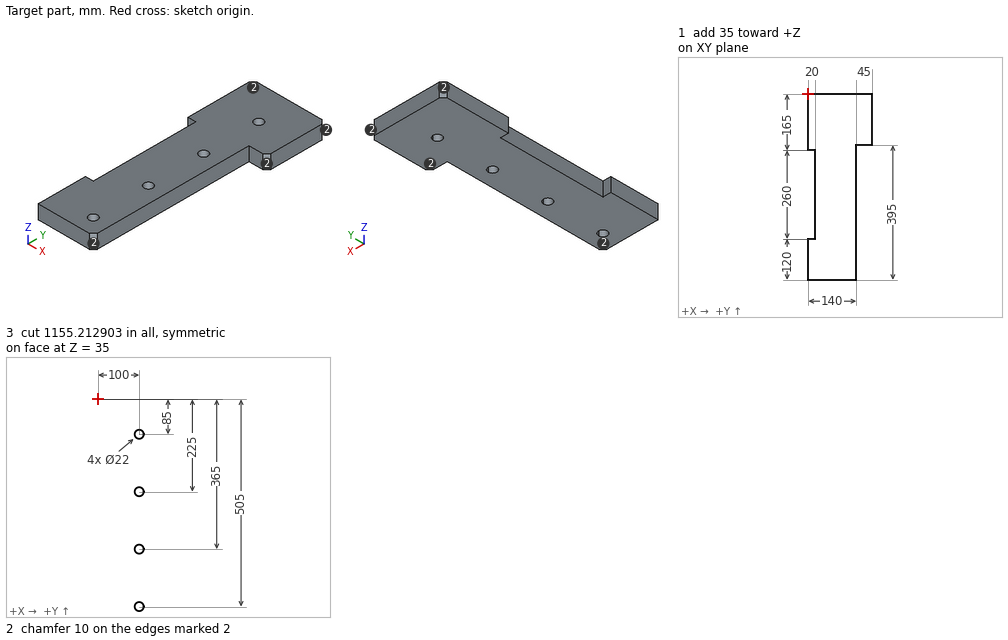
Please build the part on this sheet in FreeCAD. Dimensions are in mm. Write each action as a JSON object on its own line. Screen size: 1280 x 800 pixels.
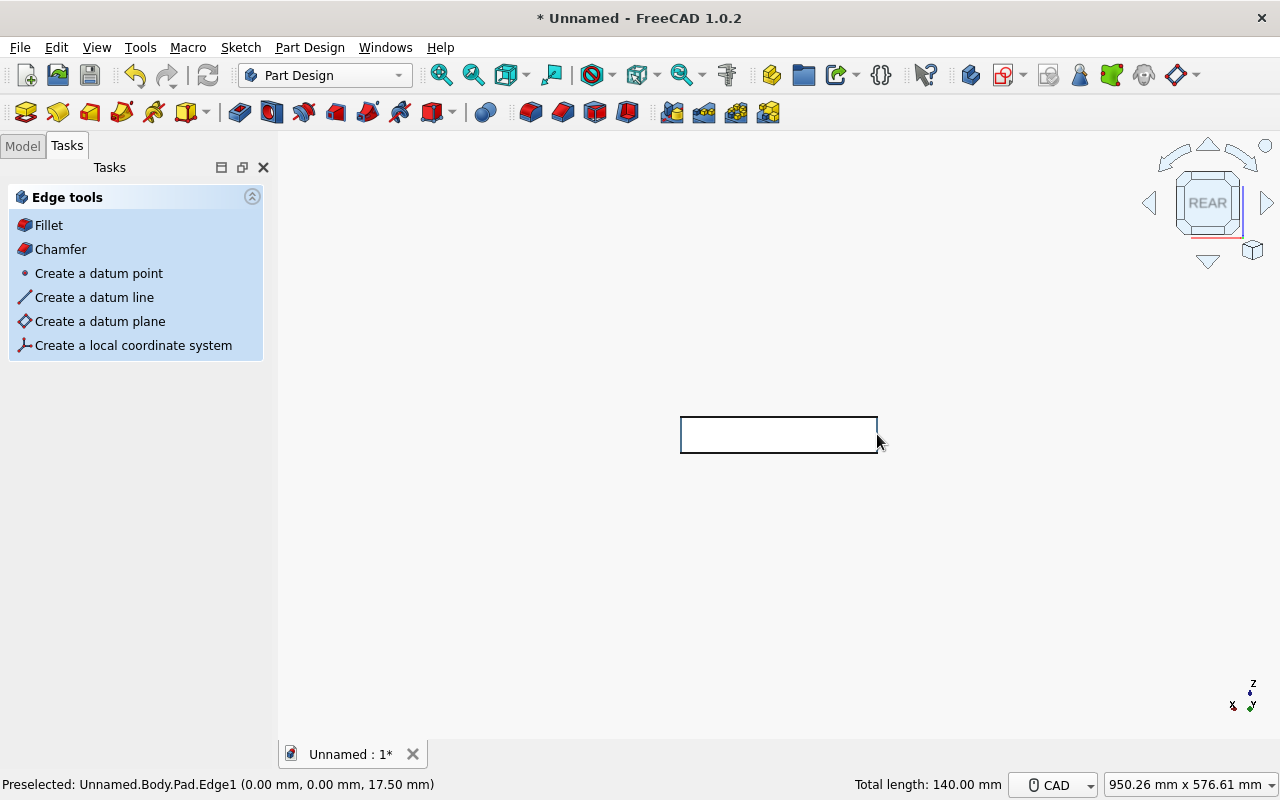
{"action": "left_click", "coordinate": [564, 112]}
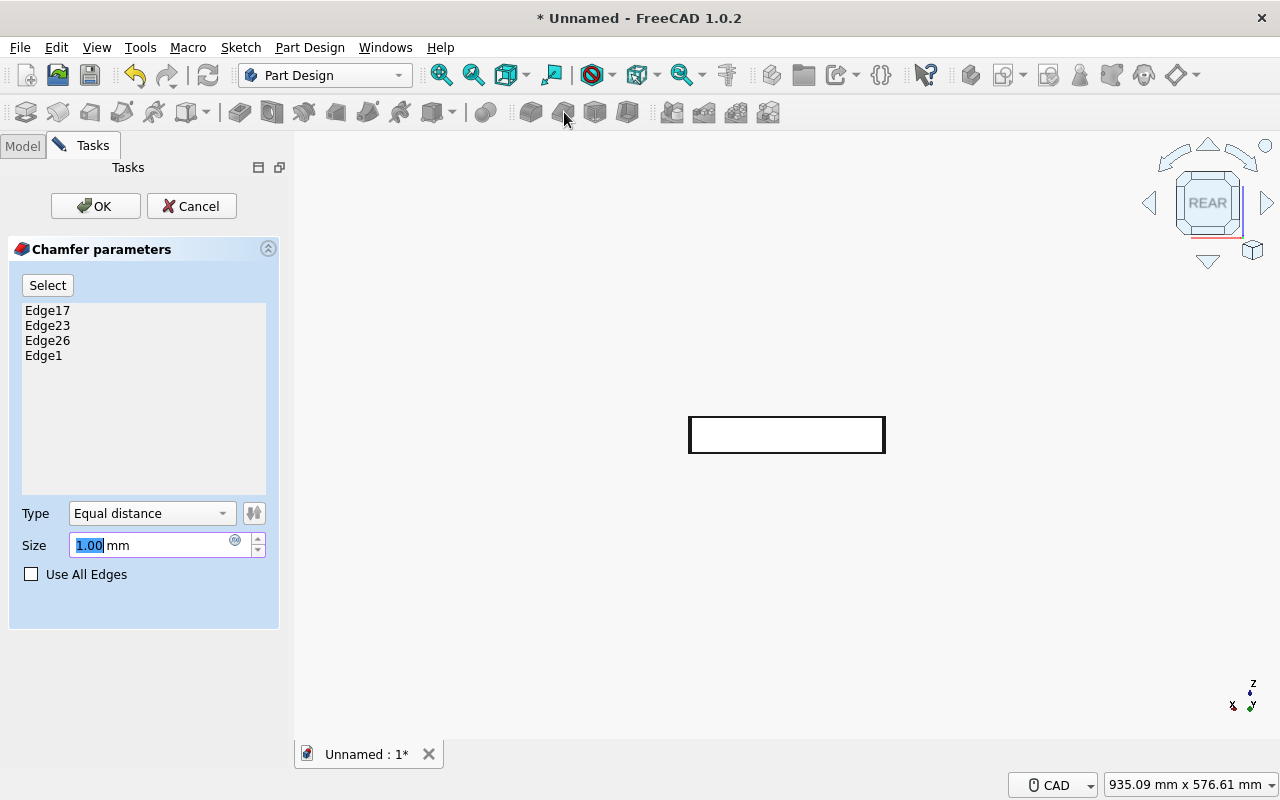
{"action": "type", "text": "10"}
{"action": "key", "text": "Tab"}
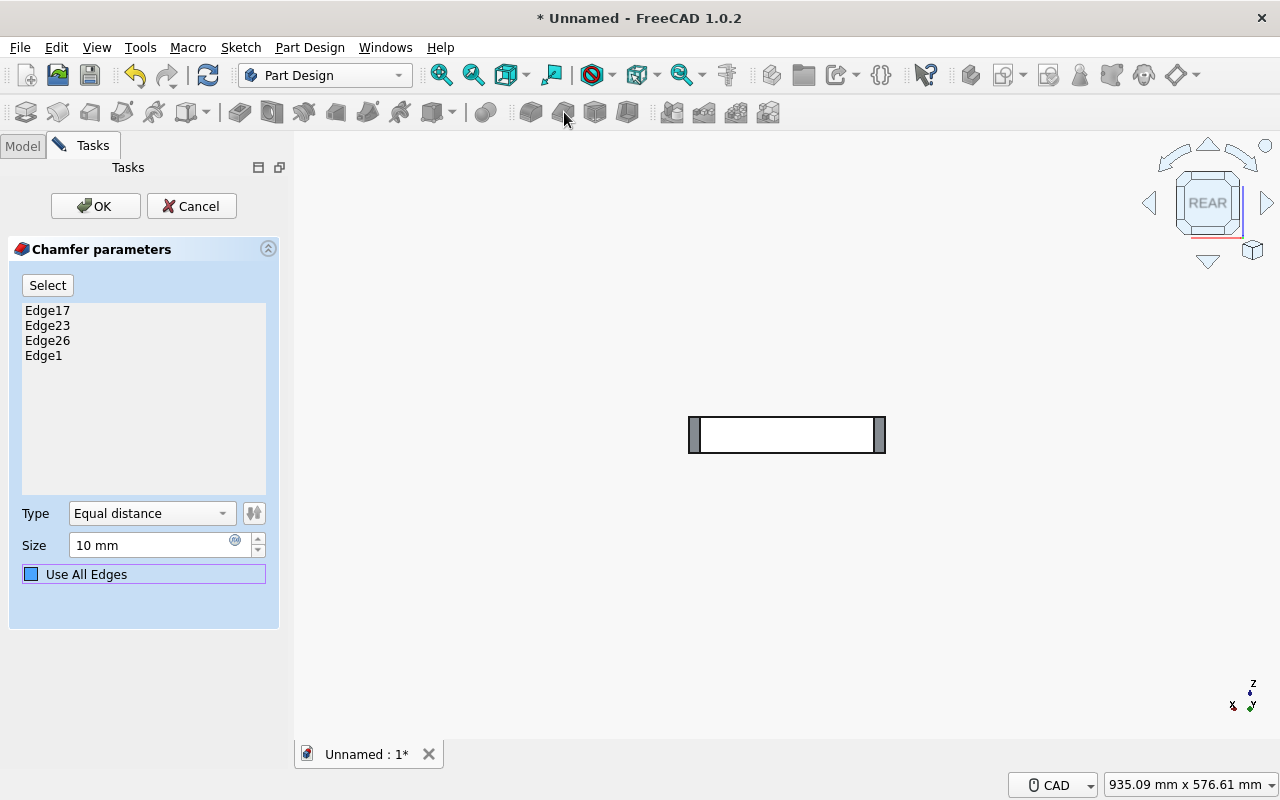
{"action": "left_click", "coordinate": [96, 206]}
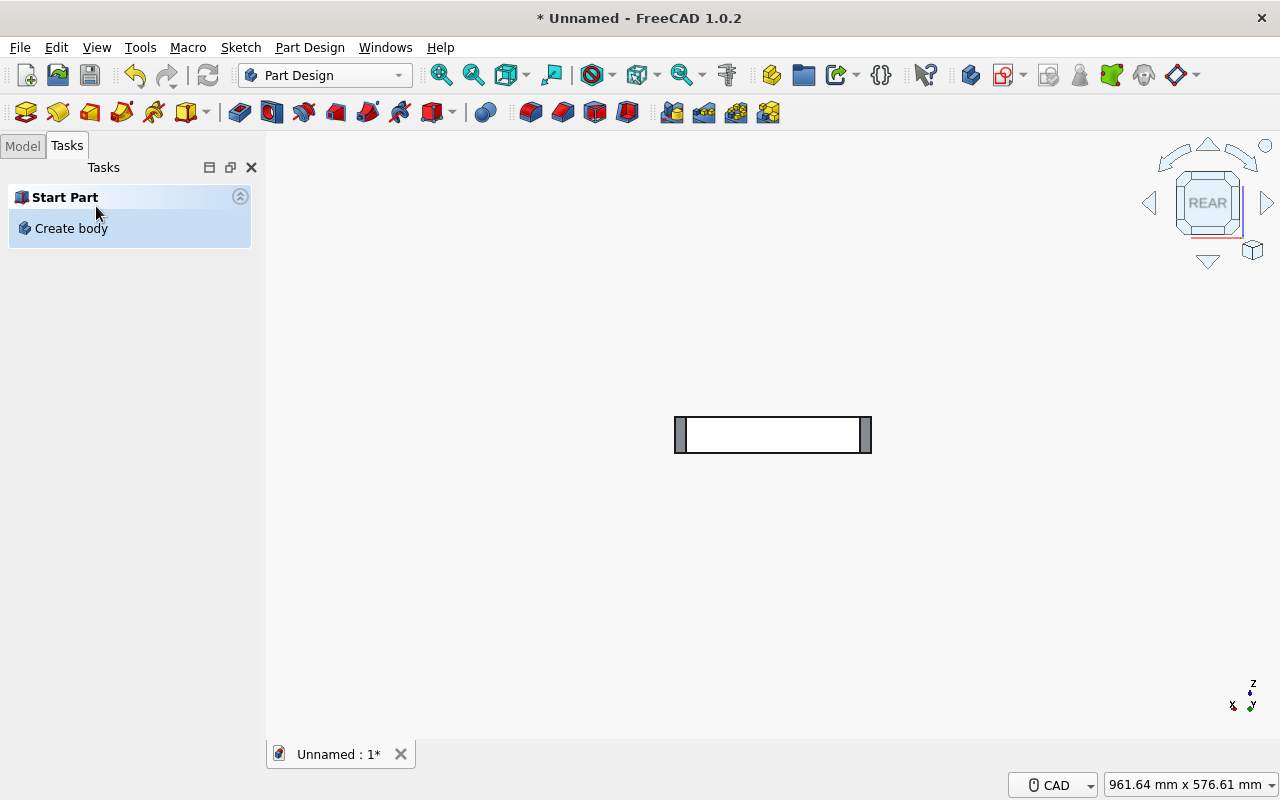
{"action": "left_click", "coordinate": [442, 76]}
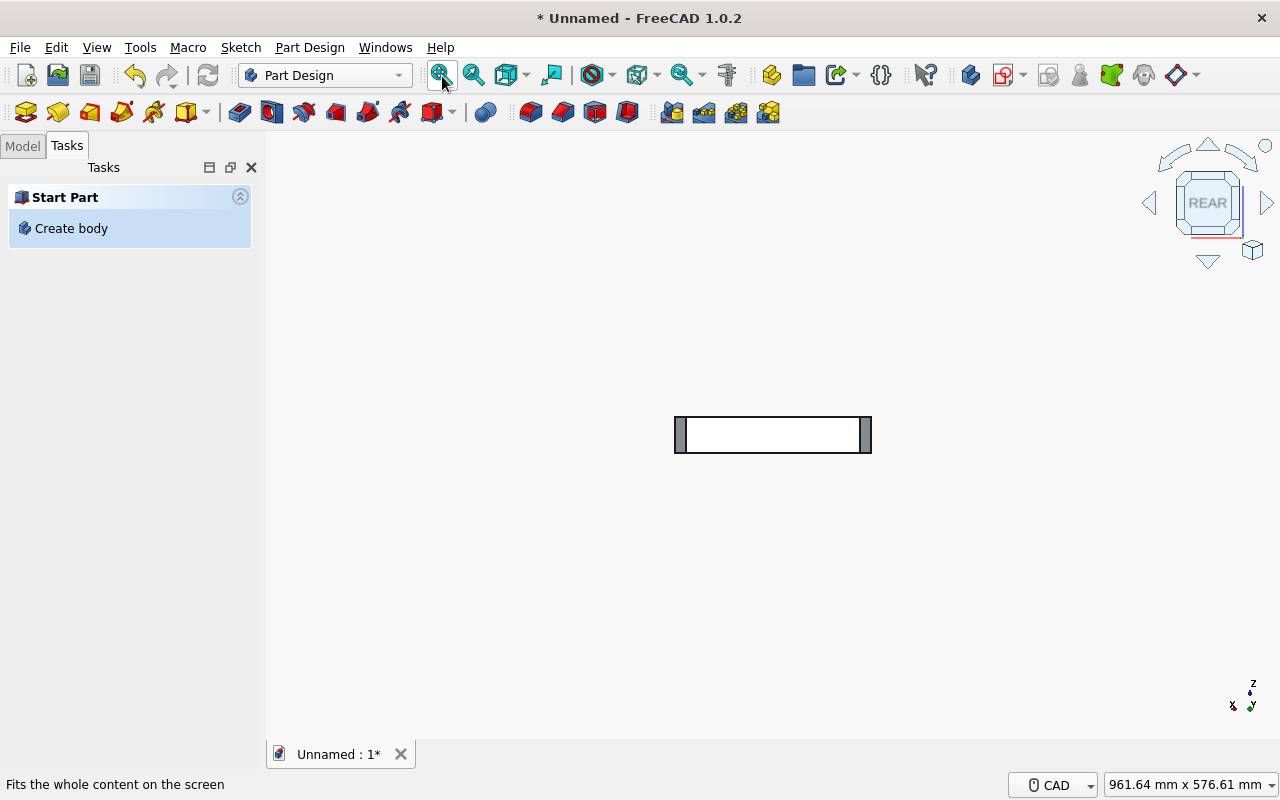
{"action": "key", "text": "0"}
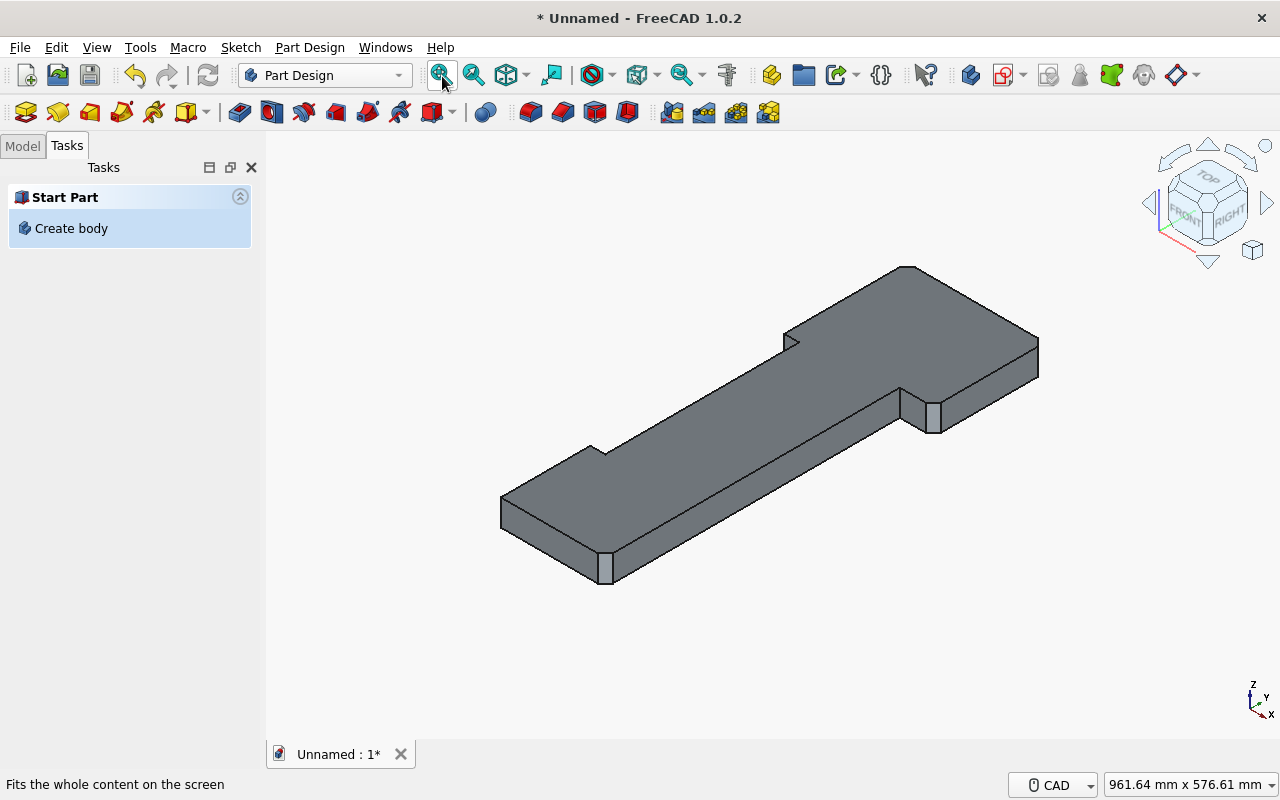
{"action": "left_click", "coordinate": [869, 341]}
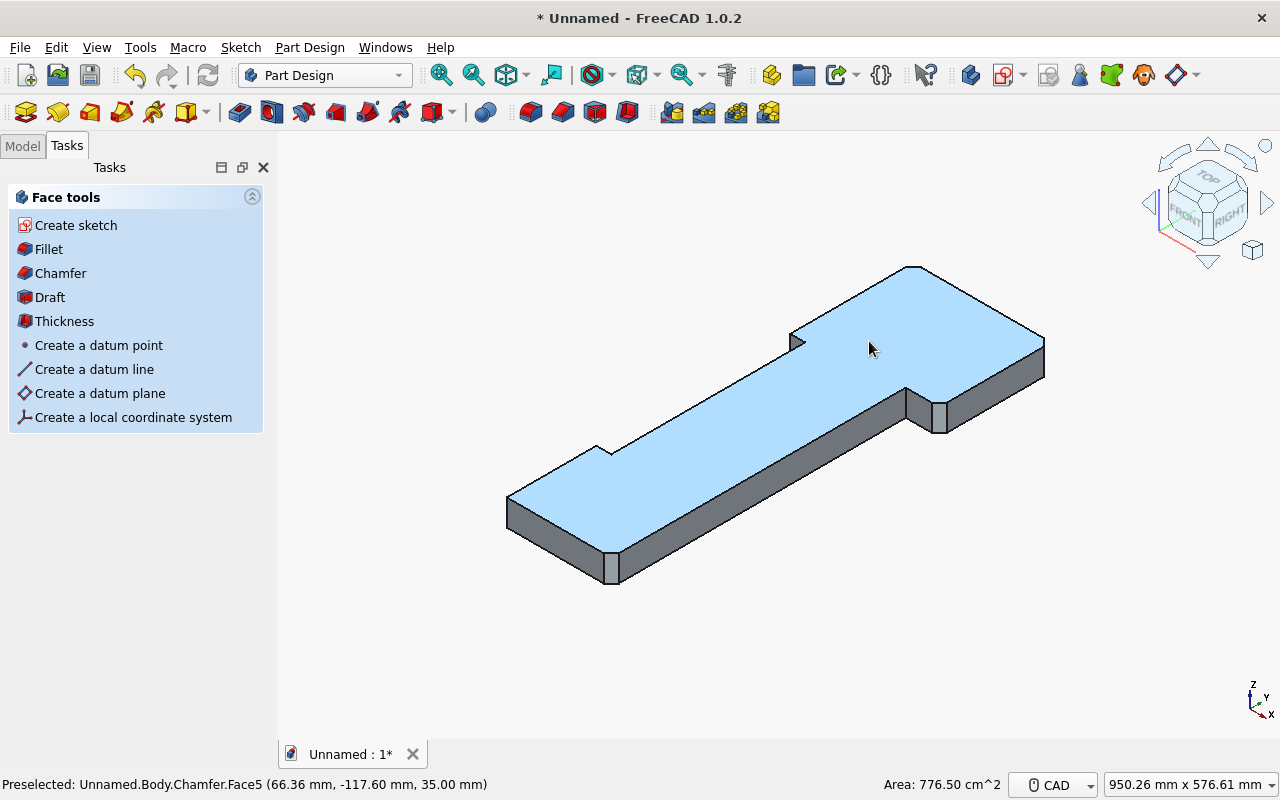
{"action": "left_click", "coordinate": [1004, 76]}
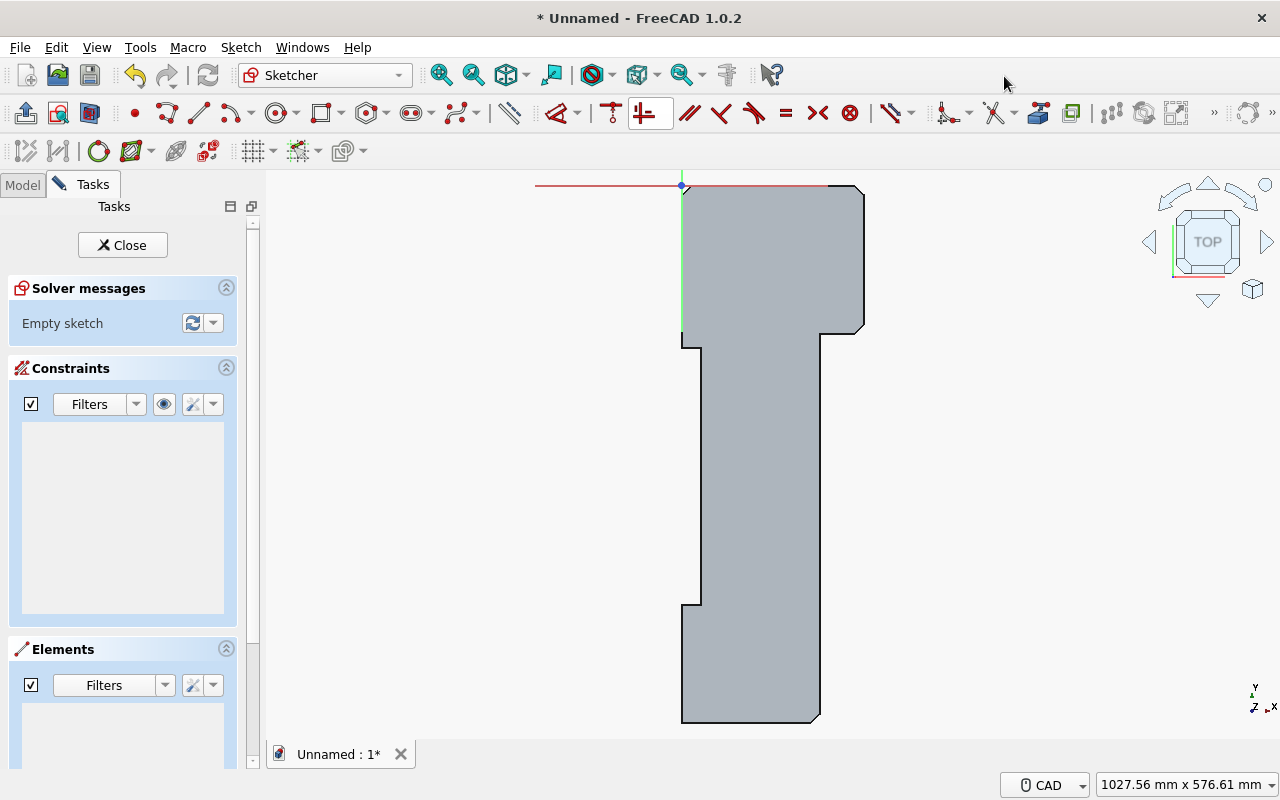
{"action": "scroll", "coordinate": [639, 484], "scroll_direction": "down", "scroll_amount": 2}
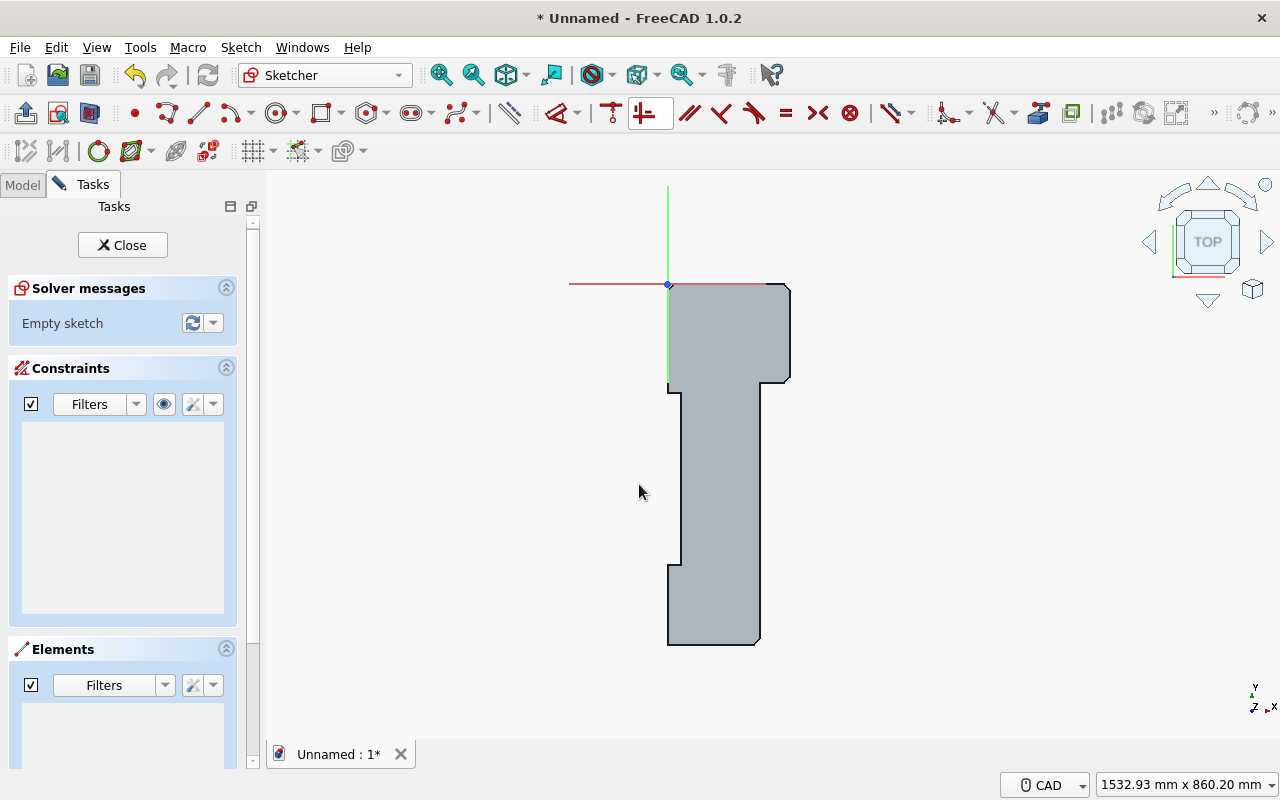
{"action": "left_click", "coordinate": [276, 114]}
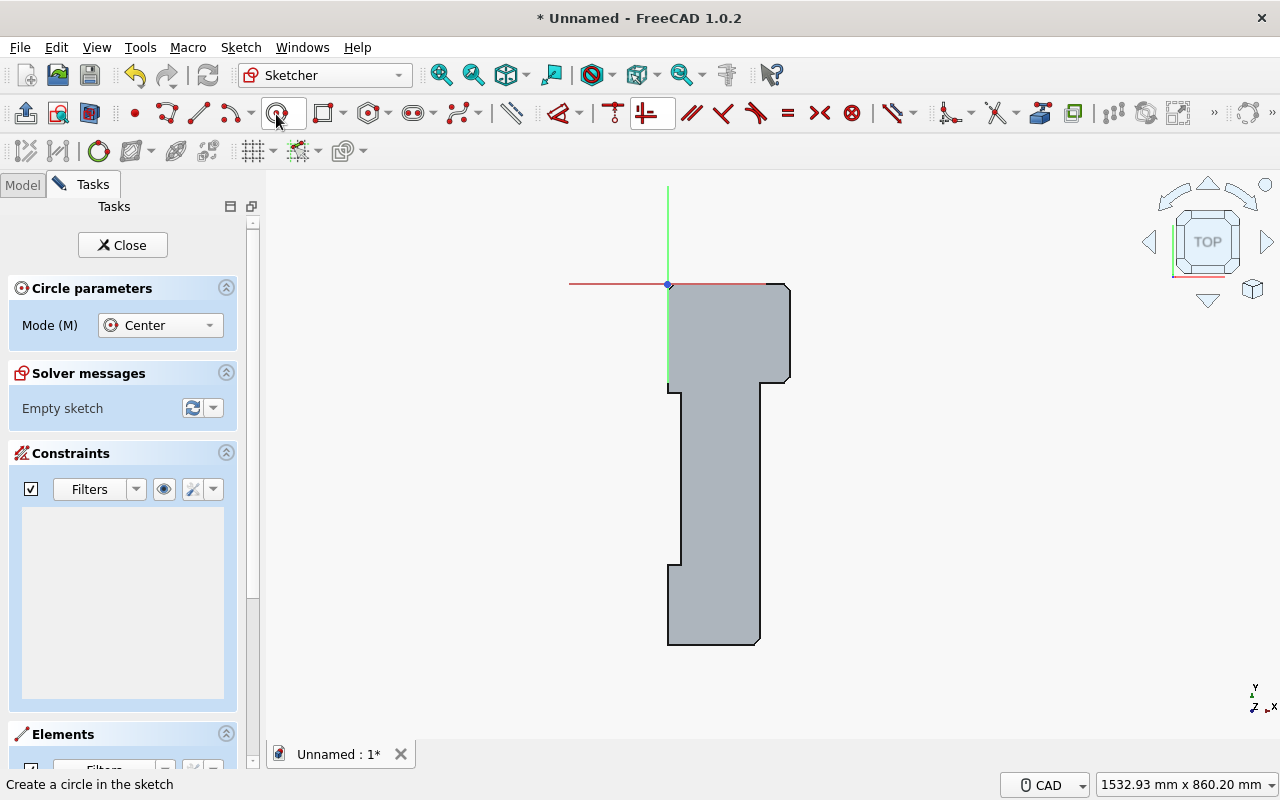
{"action": "scroll", "coordinate": [734, 340], "scroll_direction": "up", "scroll_amount": 6}